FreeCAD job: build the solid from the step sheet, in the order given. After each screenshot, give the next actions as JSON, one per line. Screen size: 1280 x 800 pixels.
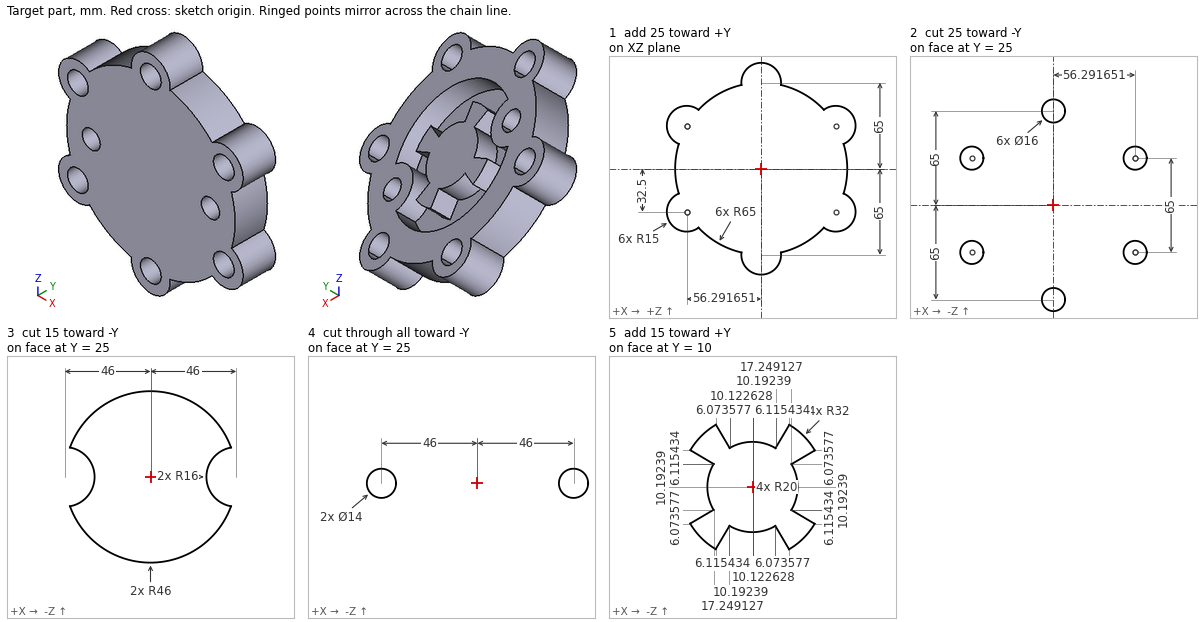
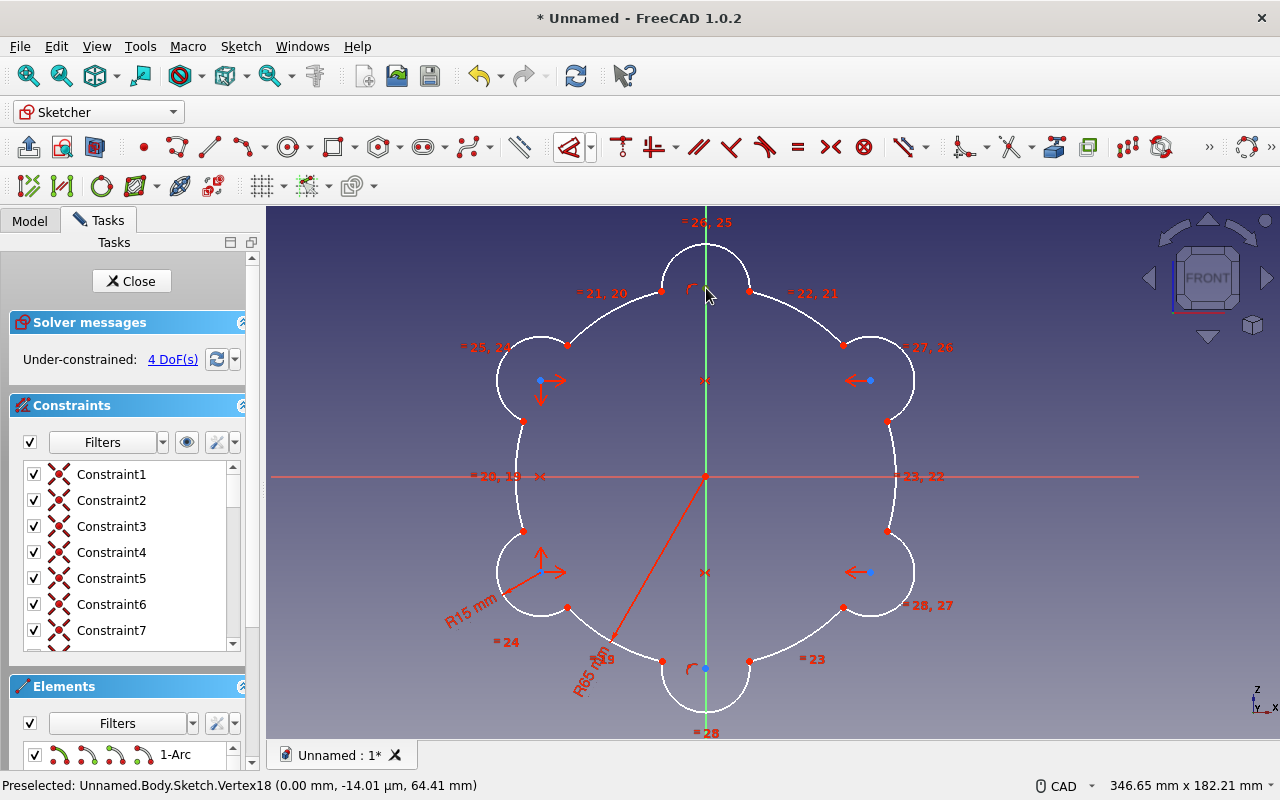
{"action": "left_click", "coordinate": [590, 148]}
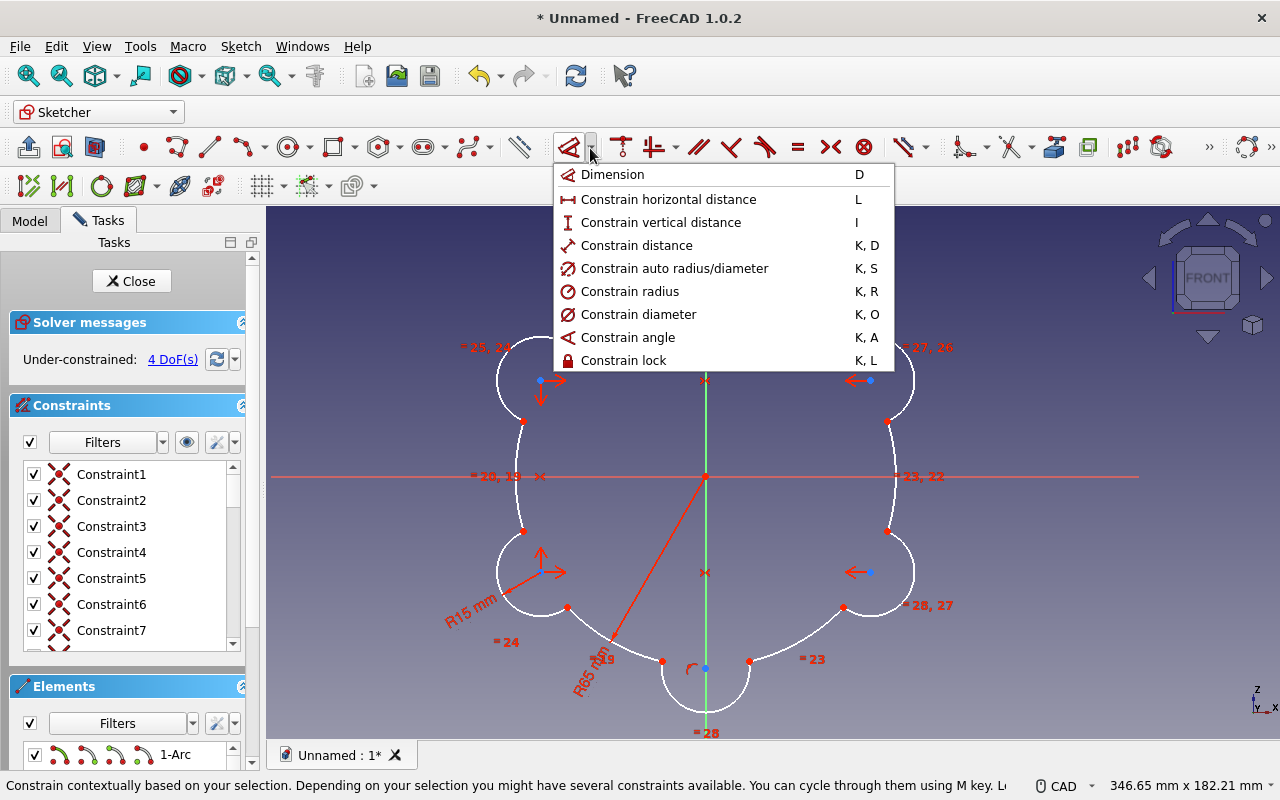
{"action": "left_click", "coordinate": [724, 222]}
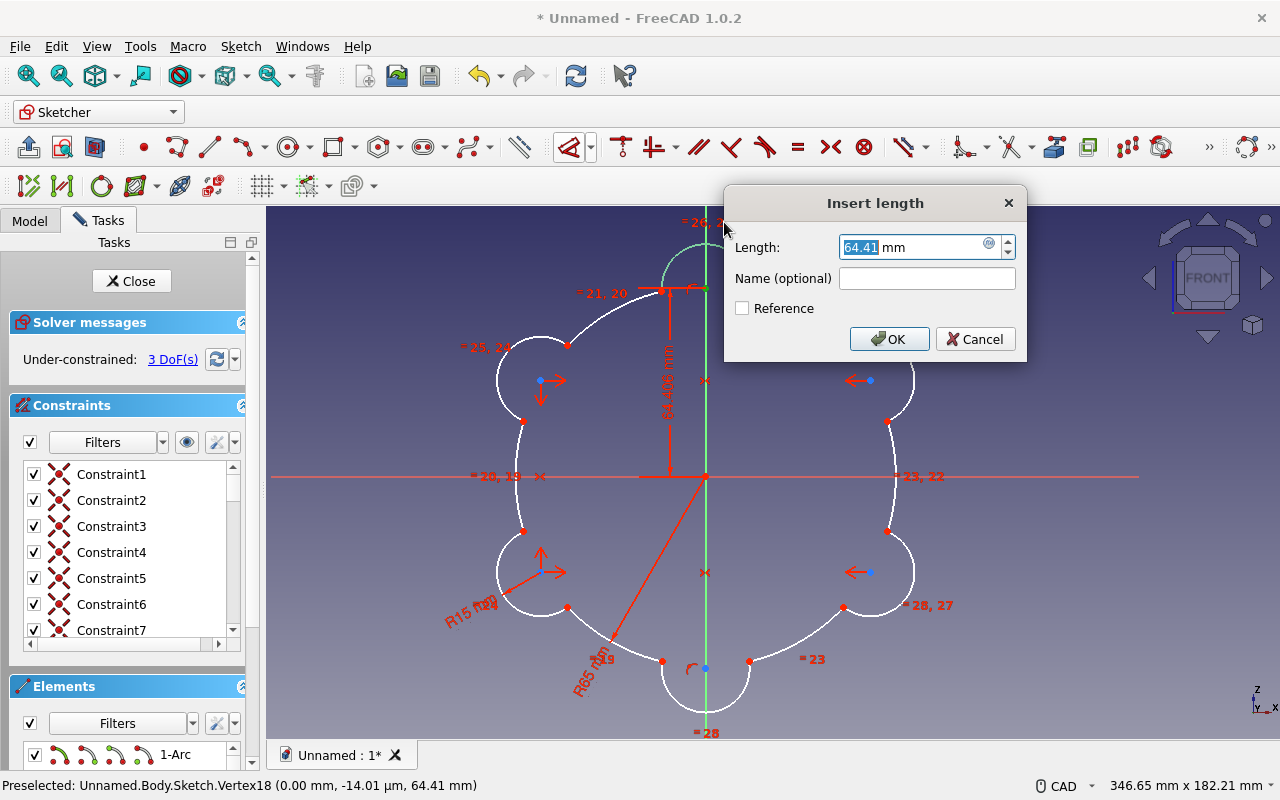
{"action": "type", "text": "65"}
{"action": "key", "text": "Return"}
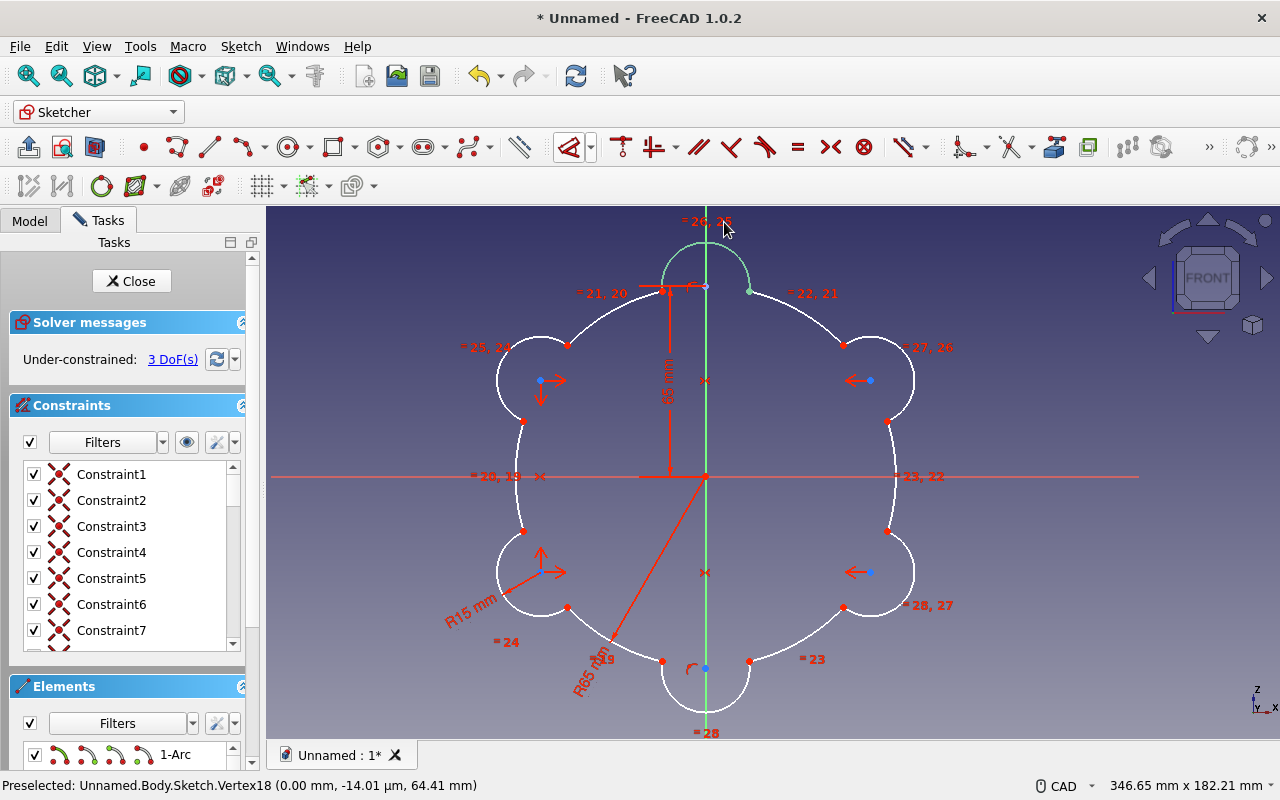
{"action": "left_click", "coordinate": [706, 669]}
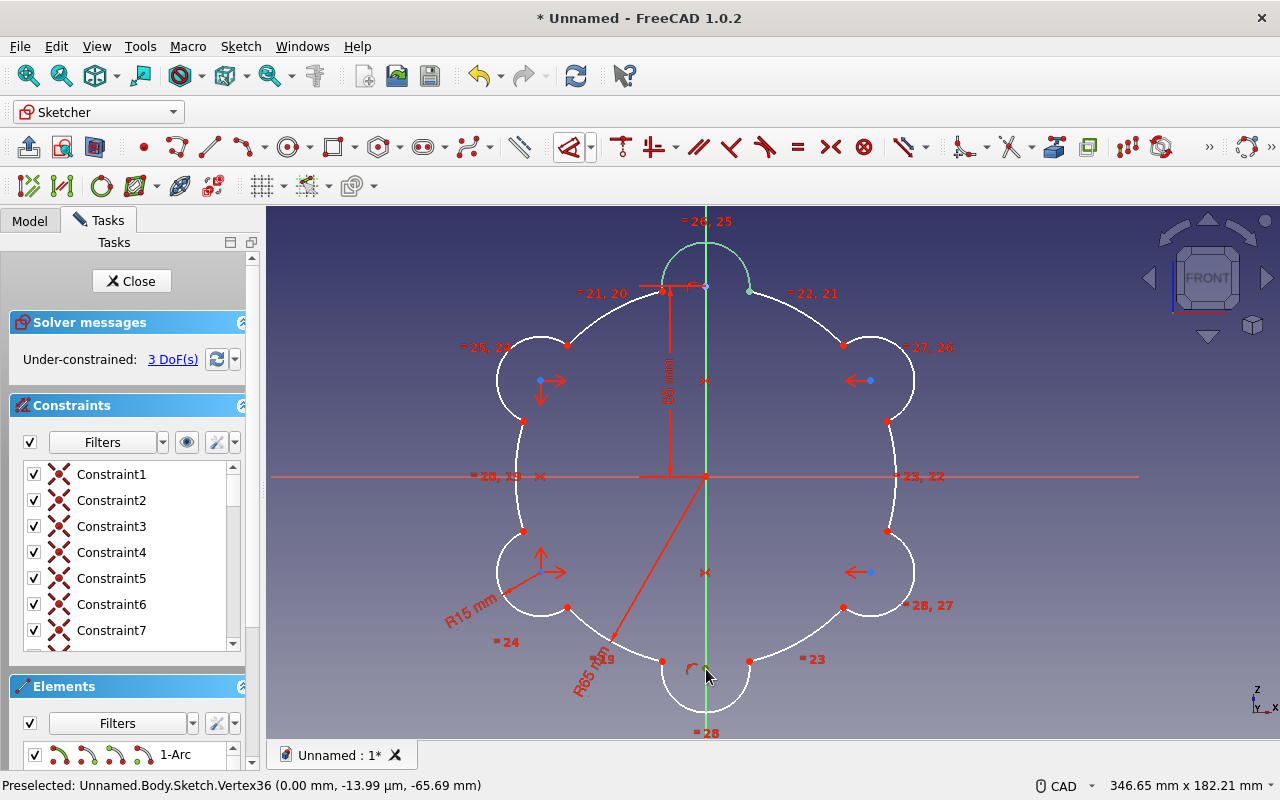
{"action": "key", "text": "i"}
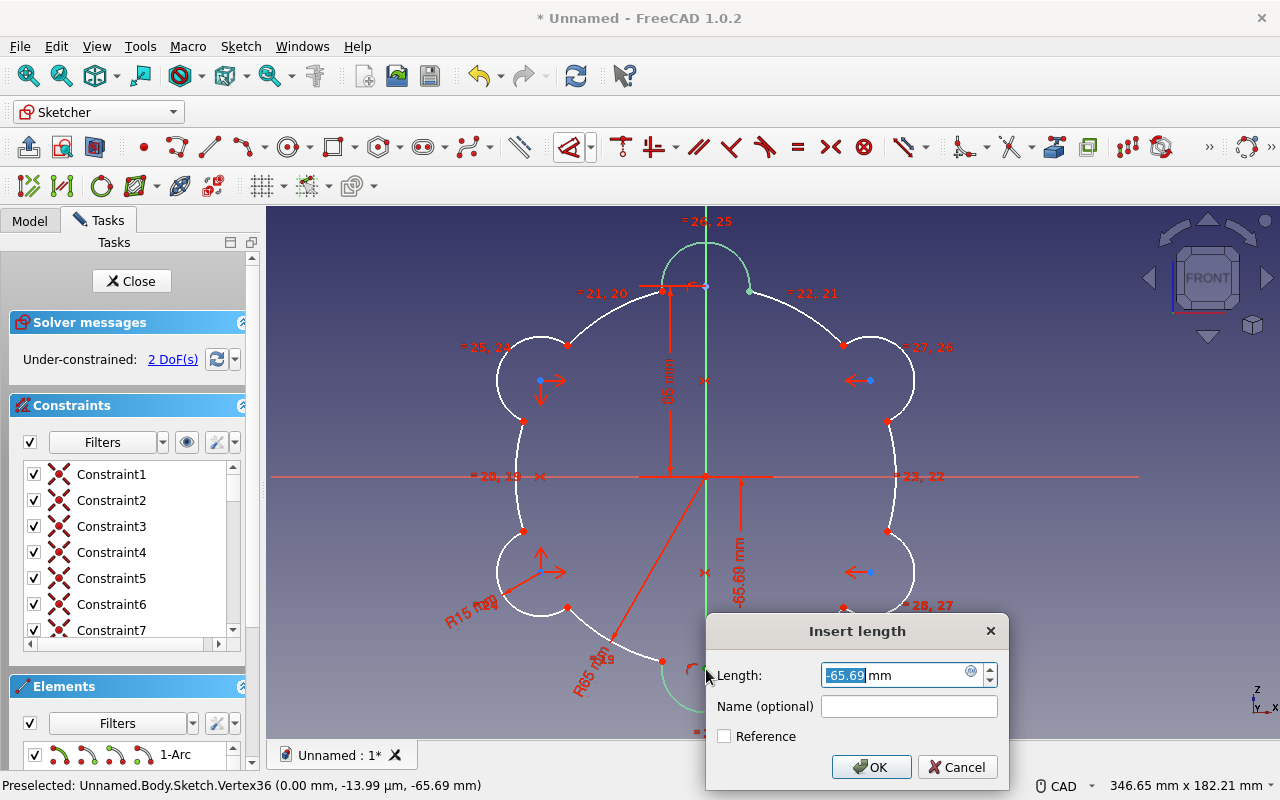
{"action": "type", "text": "-65"}
{"action": "key", "text": "Return"}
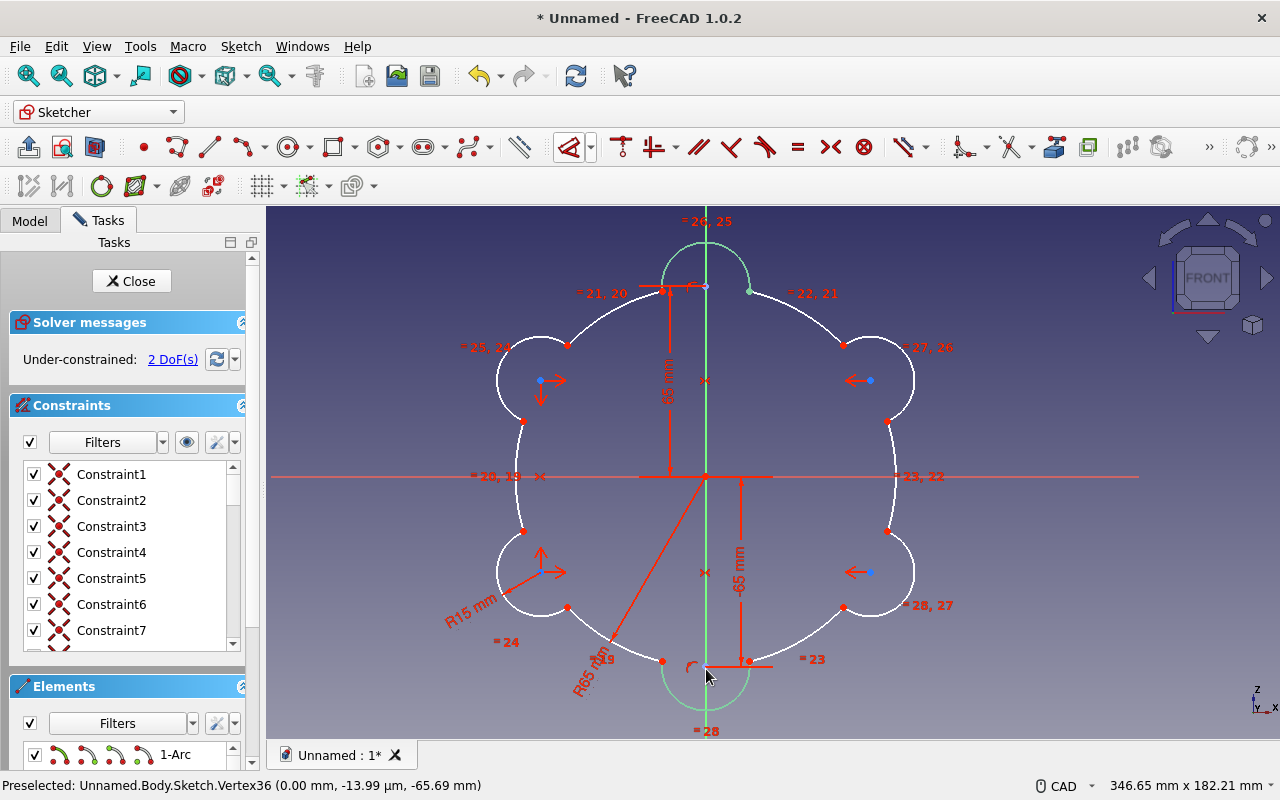
{"action": "left_click", "coordinate": [541, 572]}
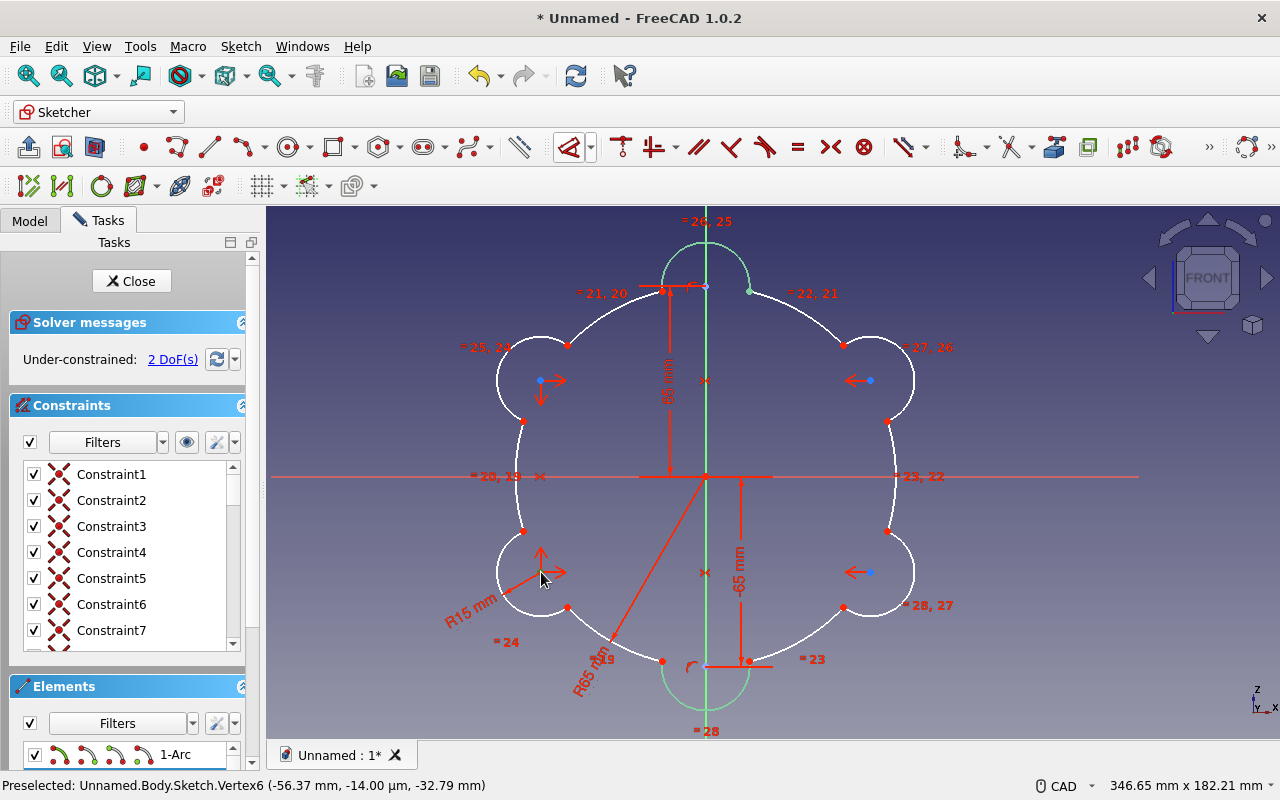
{"action": "left_click", "coordinate": [590, 148]}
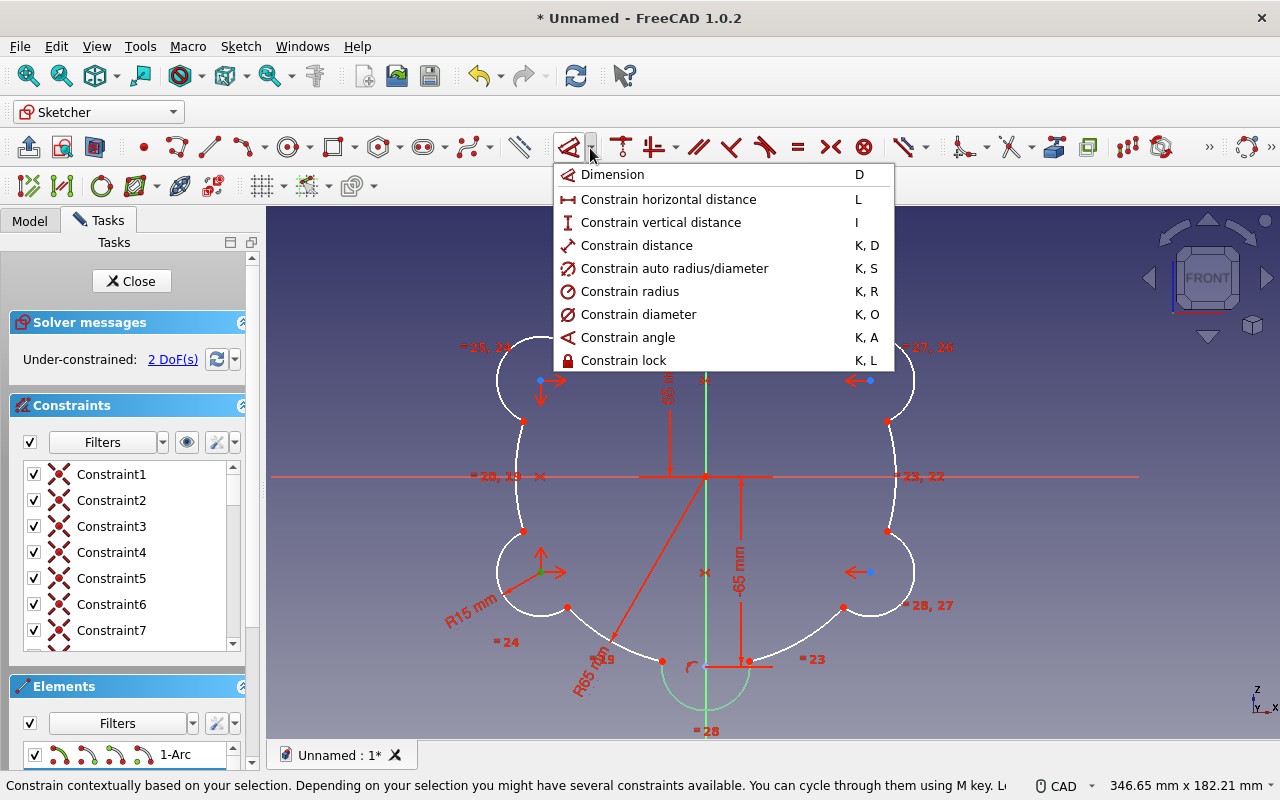
{"action": "left_click", "coordinate": [724, 222]}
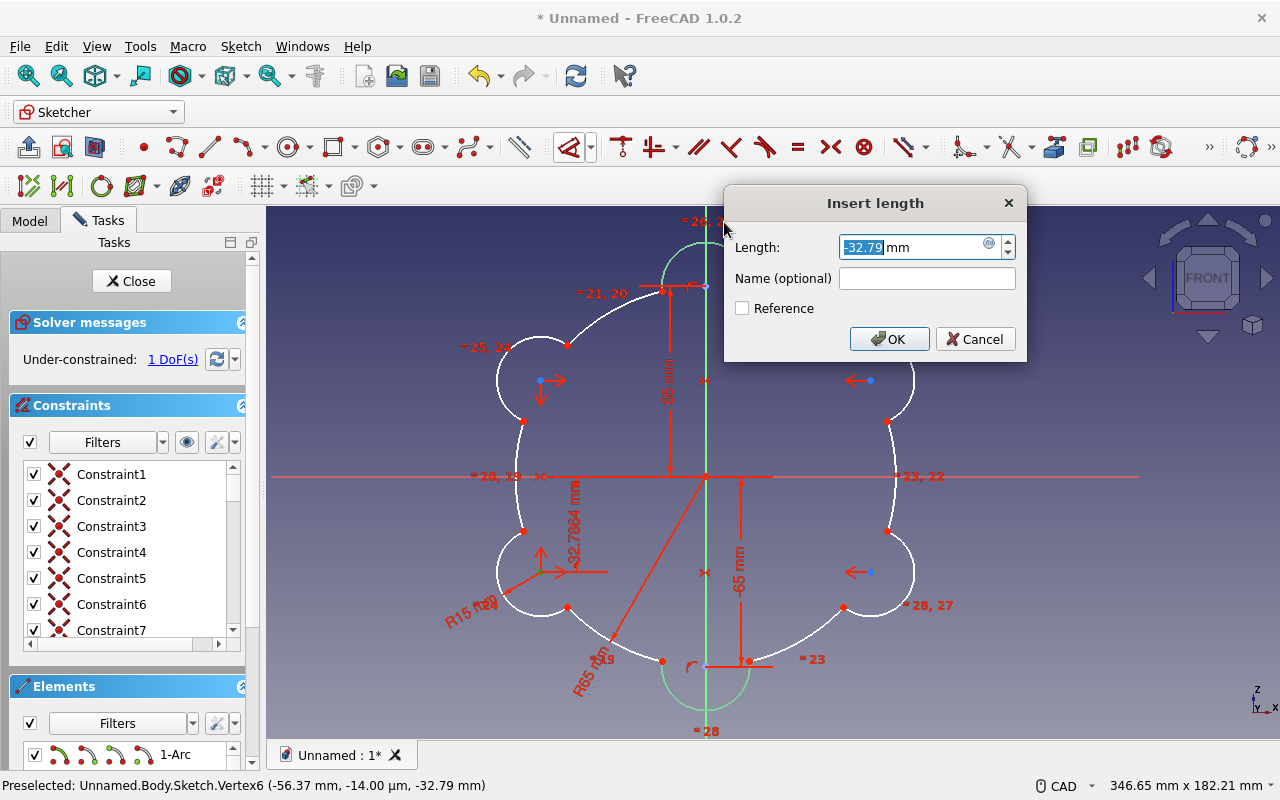
{"action": "type", "text": "-32.5"}
{"action": "key", "text": "Return"}